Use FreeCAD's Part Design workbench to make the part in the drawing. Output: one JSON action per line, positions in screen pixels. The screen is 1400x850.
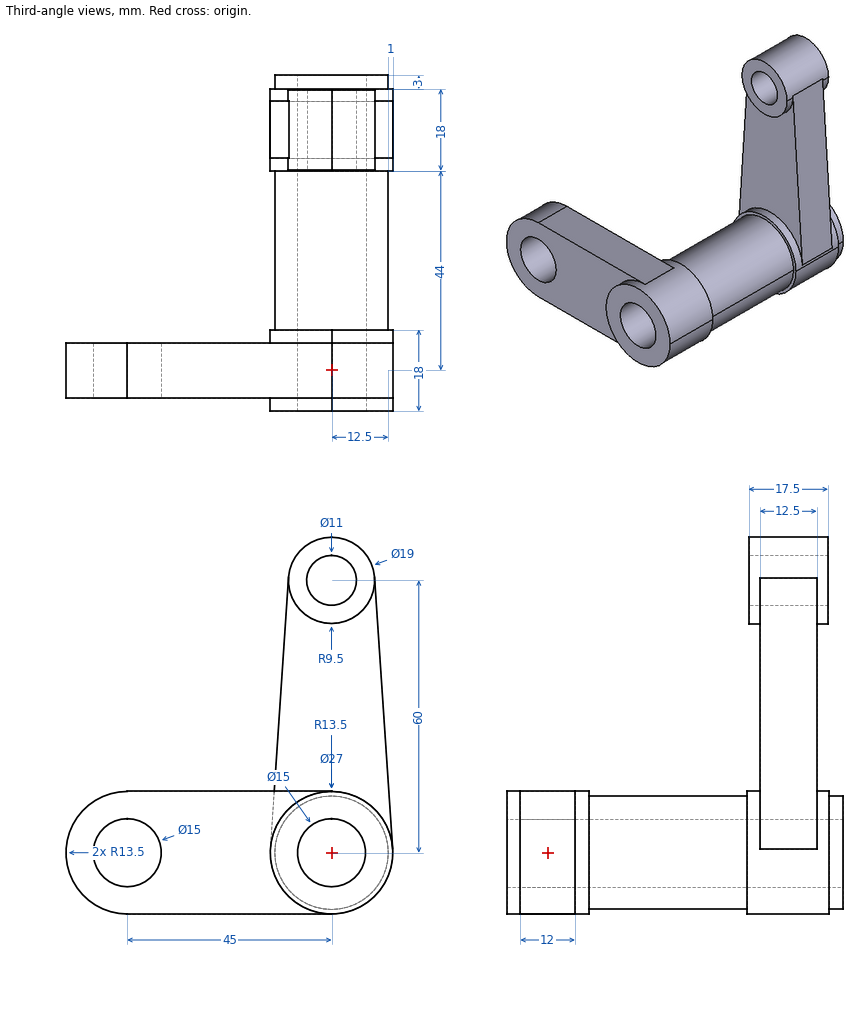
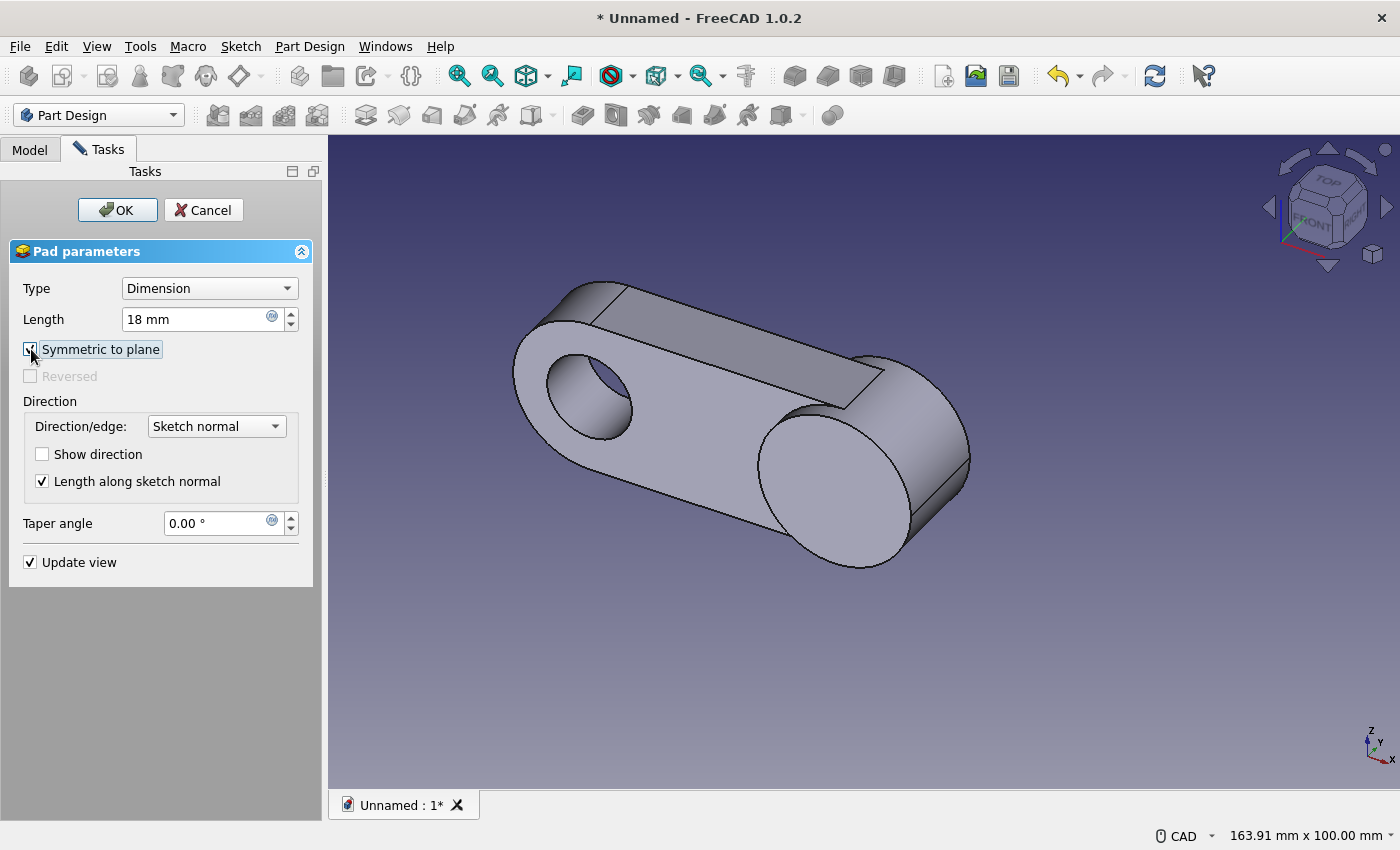
{"action": "left_click", "coordinate": [118, 210]}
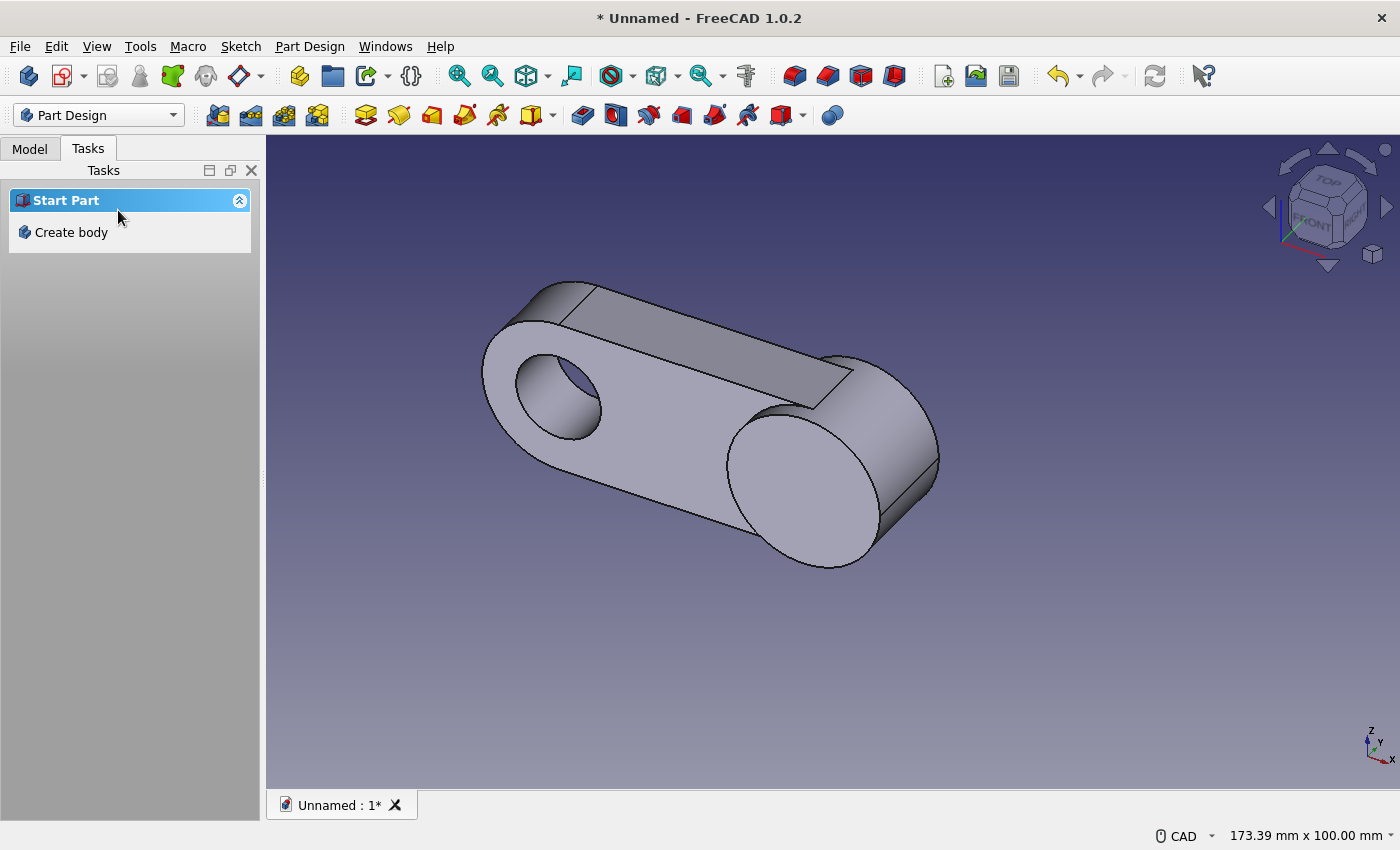
{"action": "left_click", "coordinate": [62, 76]}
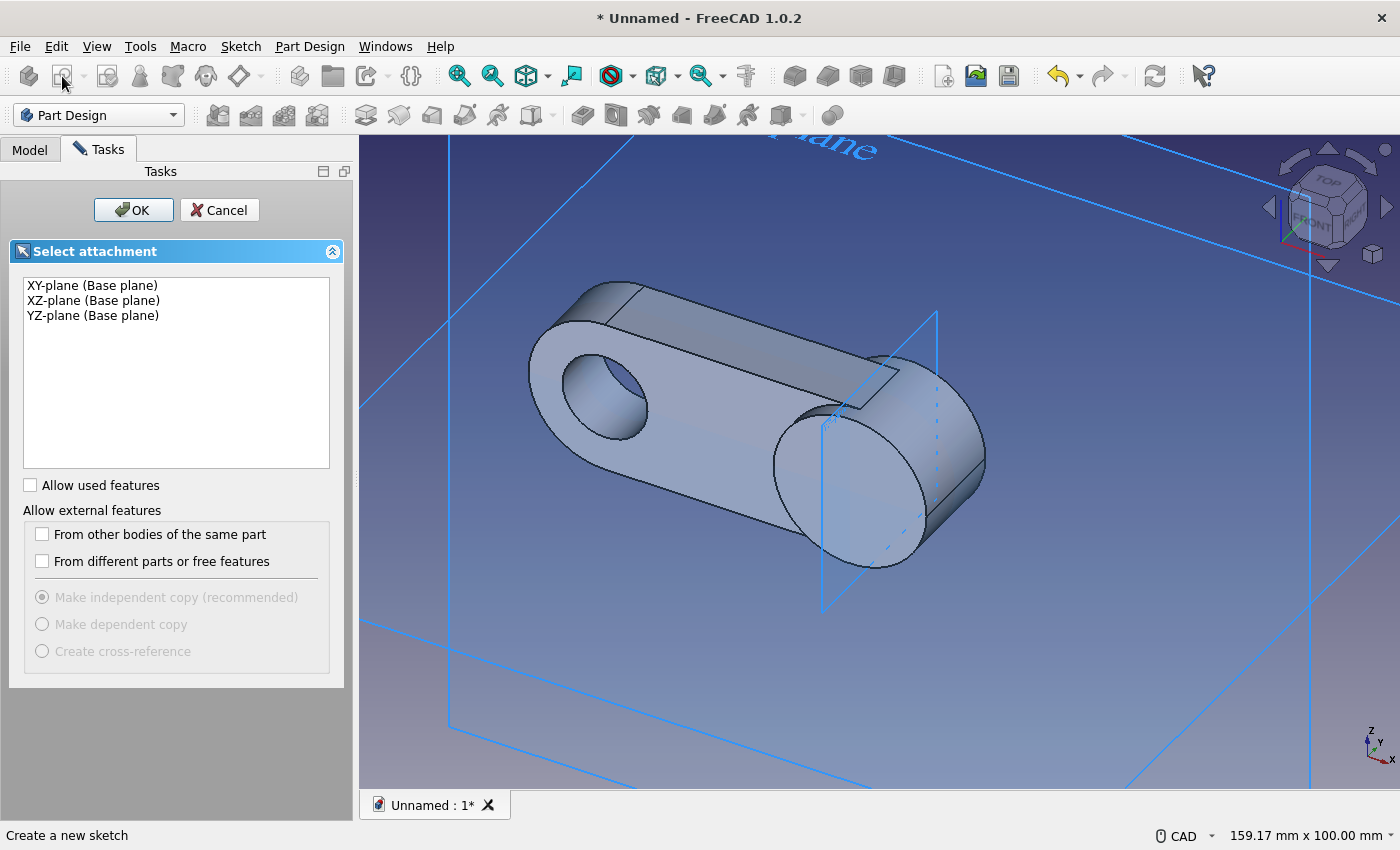
{"action": "left_click", "coordinate": [84, 286]}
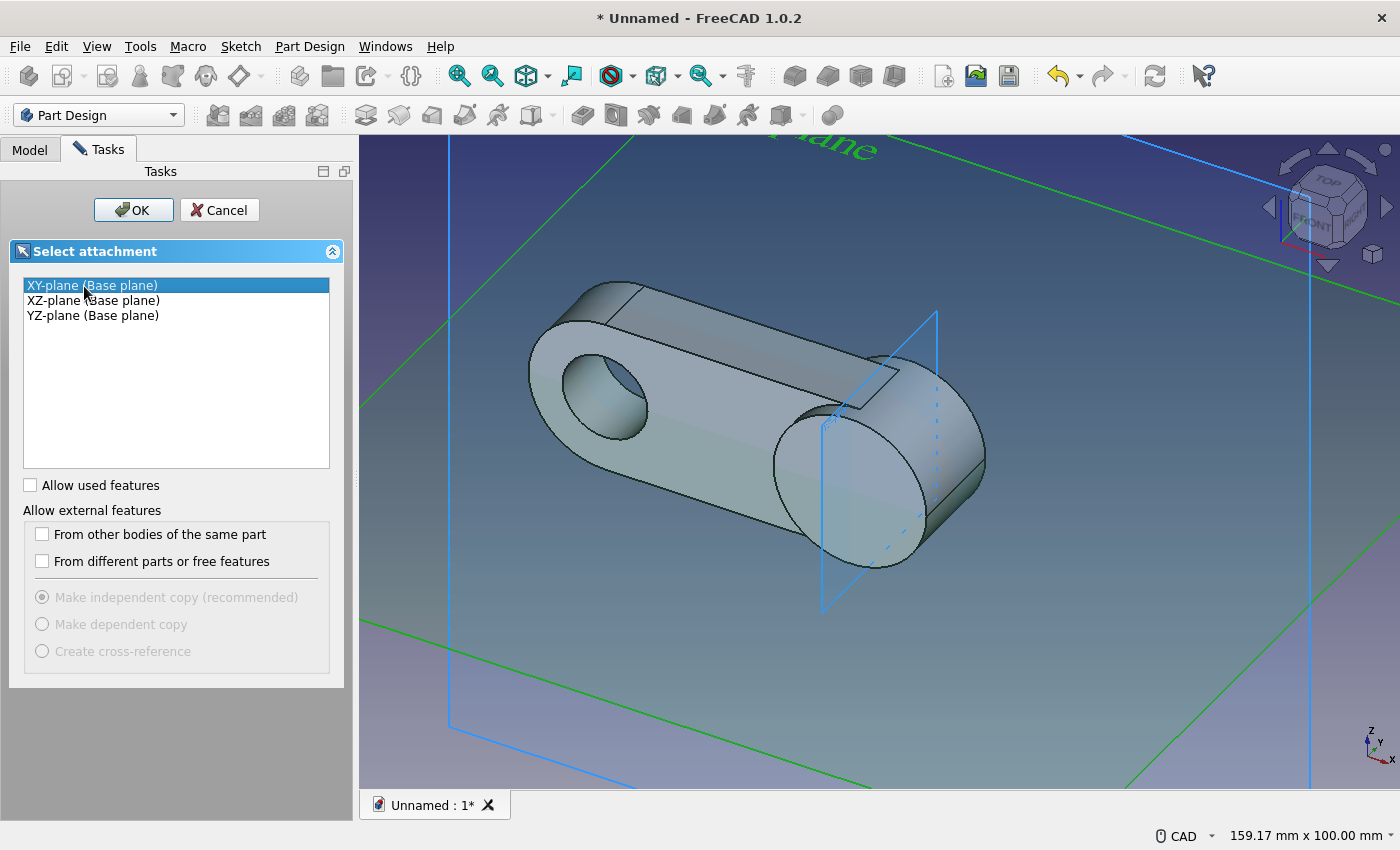
{"action": "left_click", "coordinate": [134, 210]}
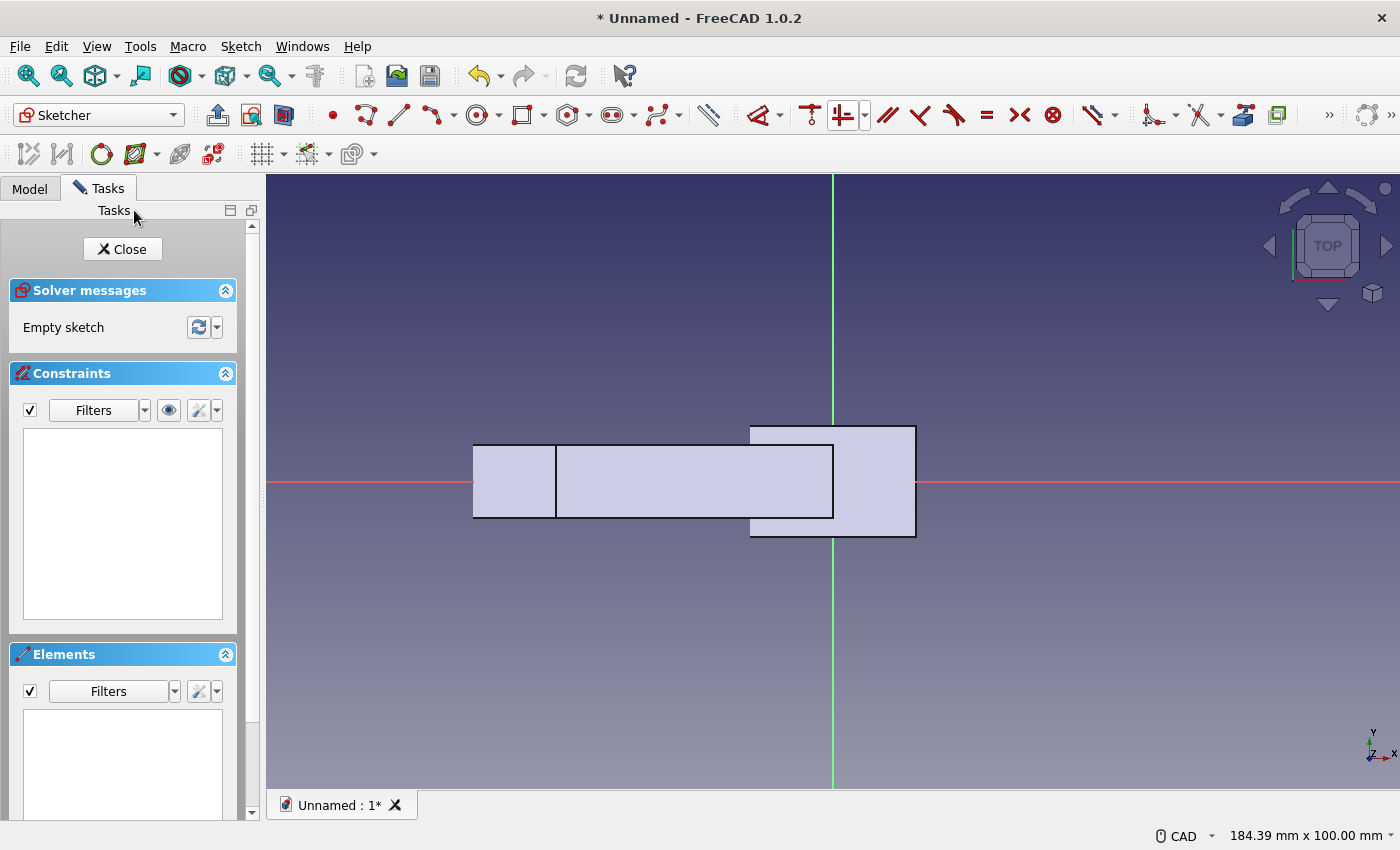
{"action": "key", "text": "q s"}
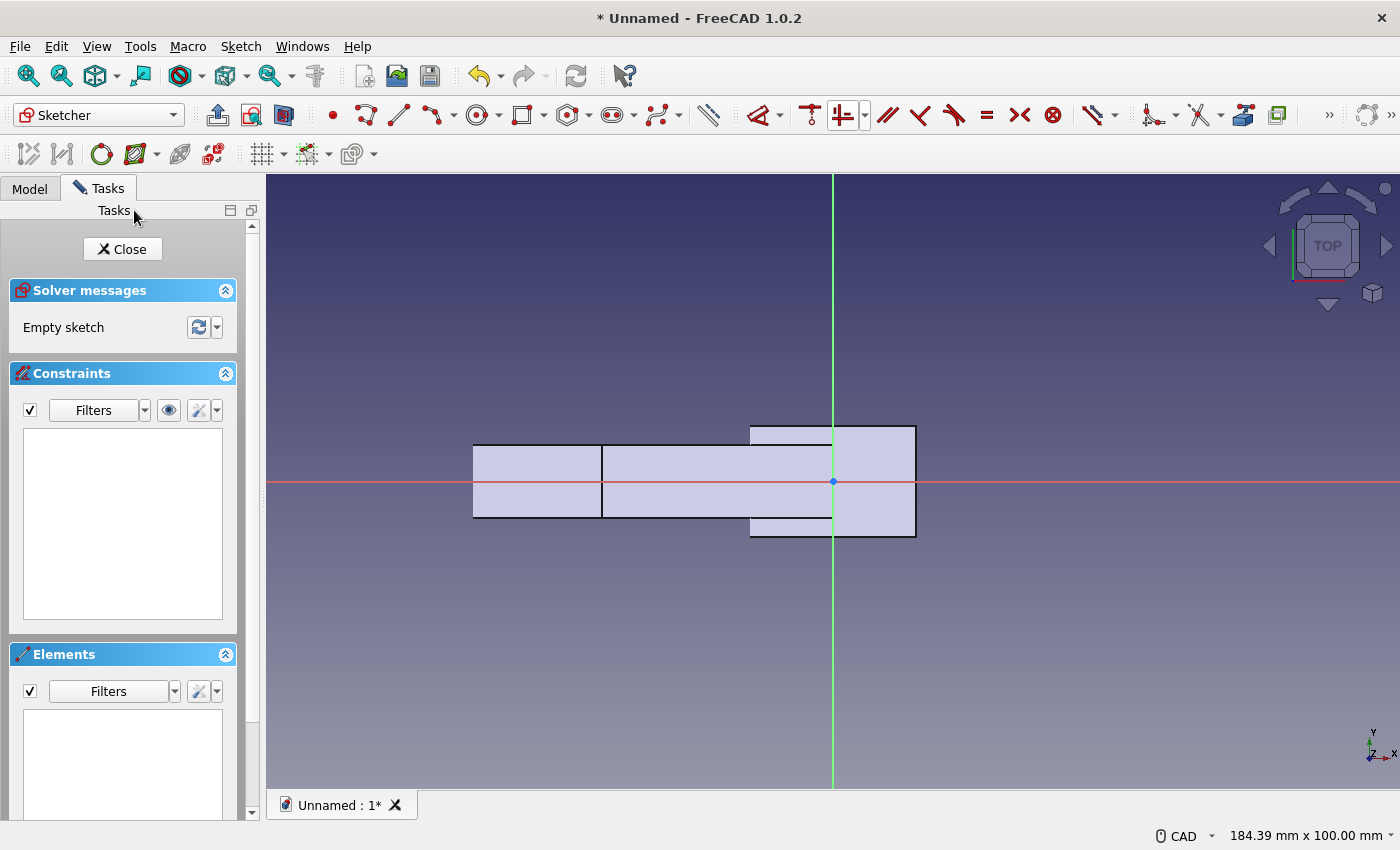
{"action": "scroll", "coordinate": [541, 761], "scroll_direction": "down", "scroll_amount": 2}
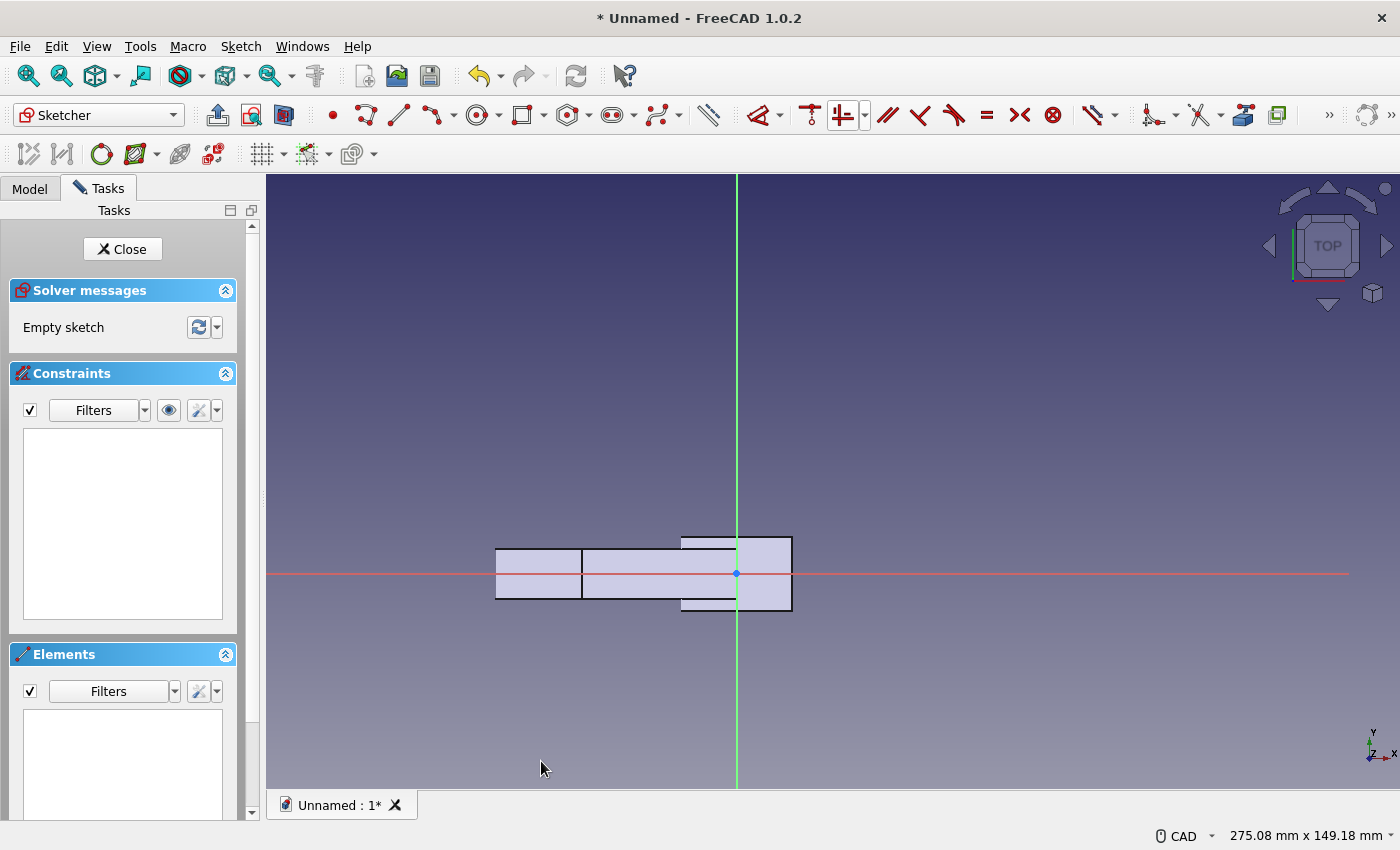
{"action": "scroll", "coordinate": [765, 356], "scroll_direction": "up", "scroll_amount": 2}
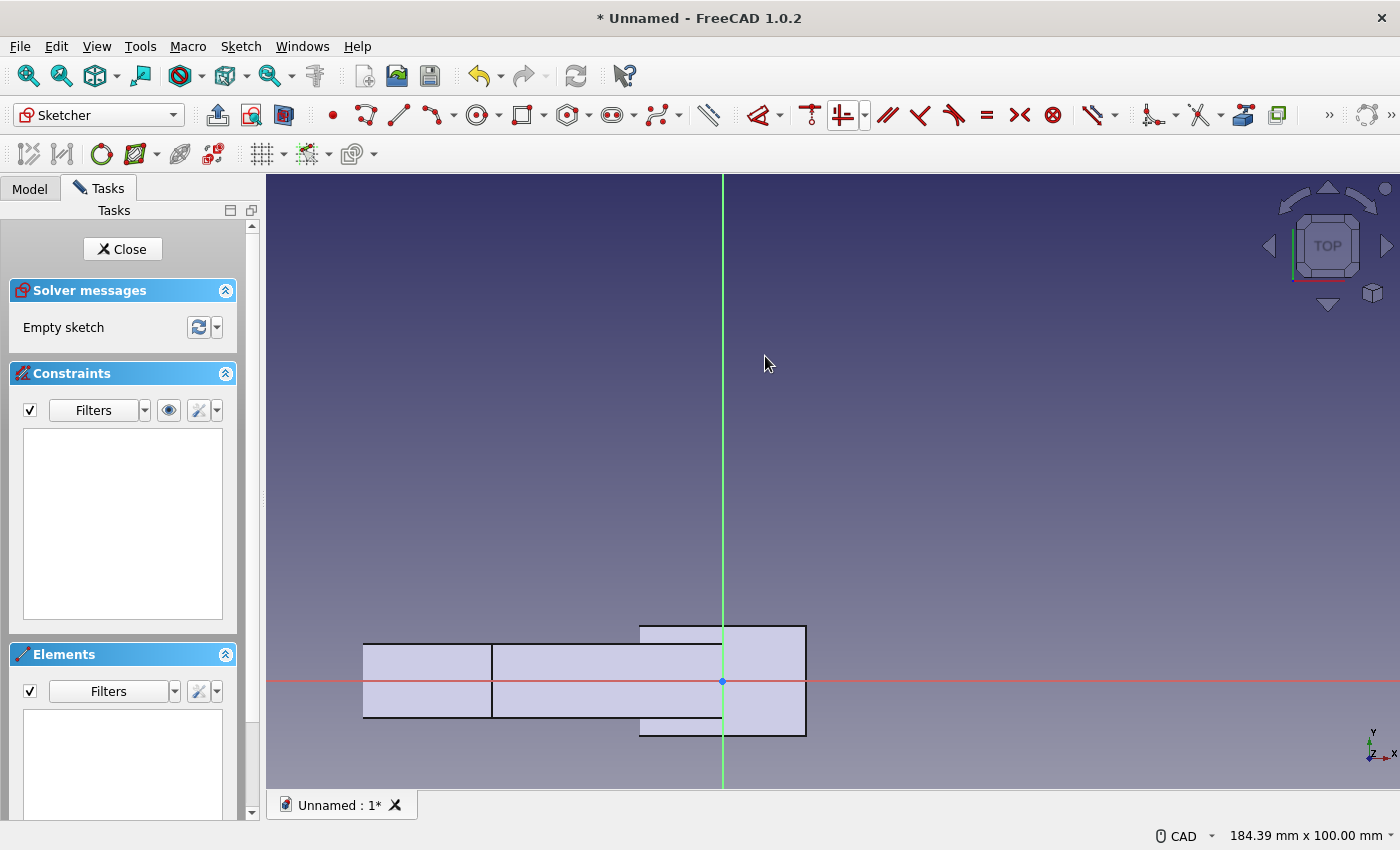
{"action": "left_click", "coordinate": [366, 116]}